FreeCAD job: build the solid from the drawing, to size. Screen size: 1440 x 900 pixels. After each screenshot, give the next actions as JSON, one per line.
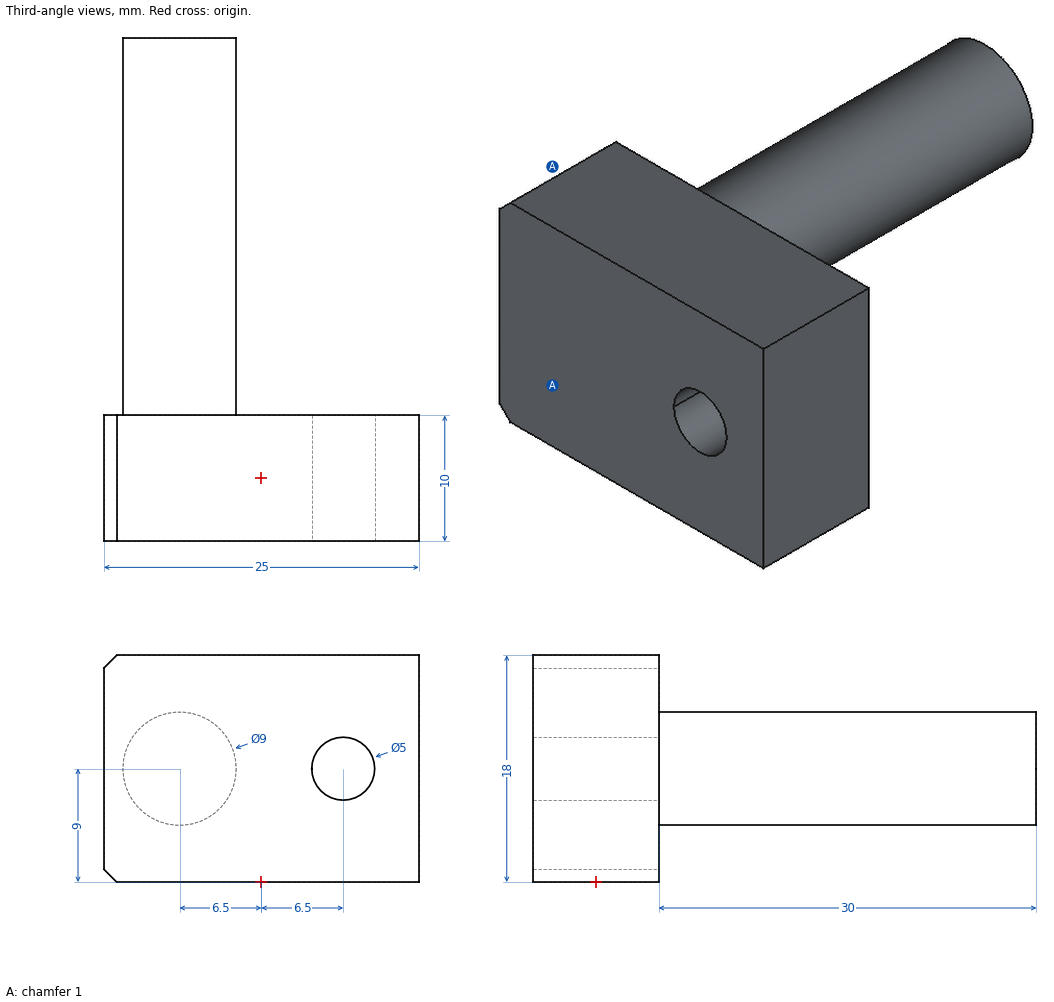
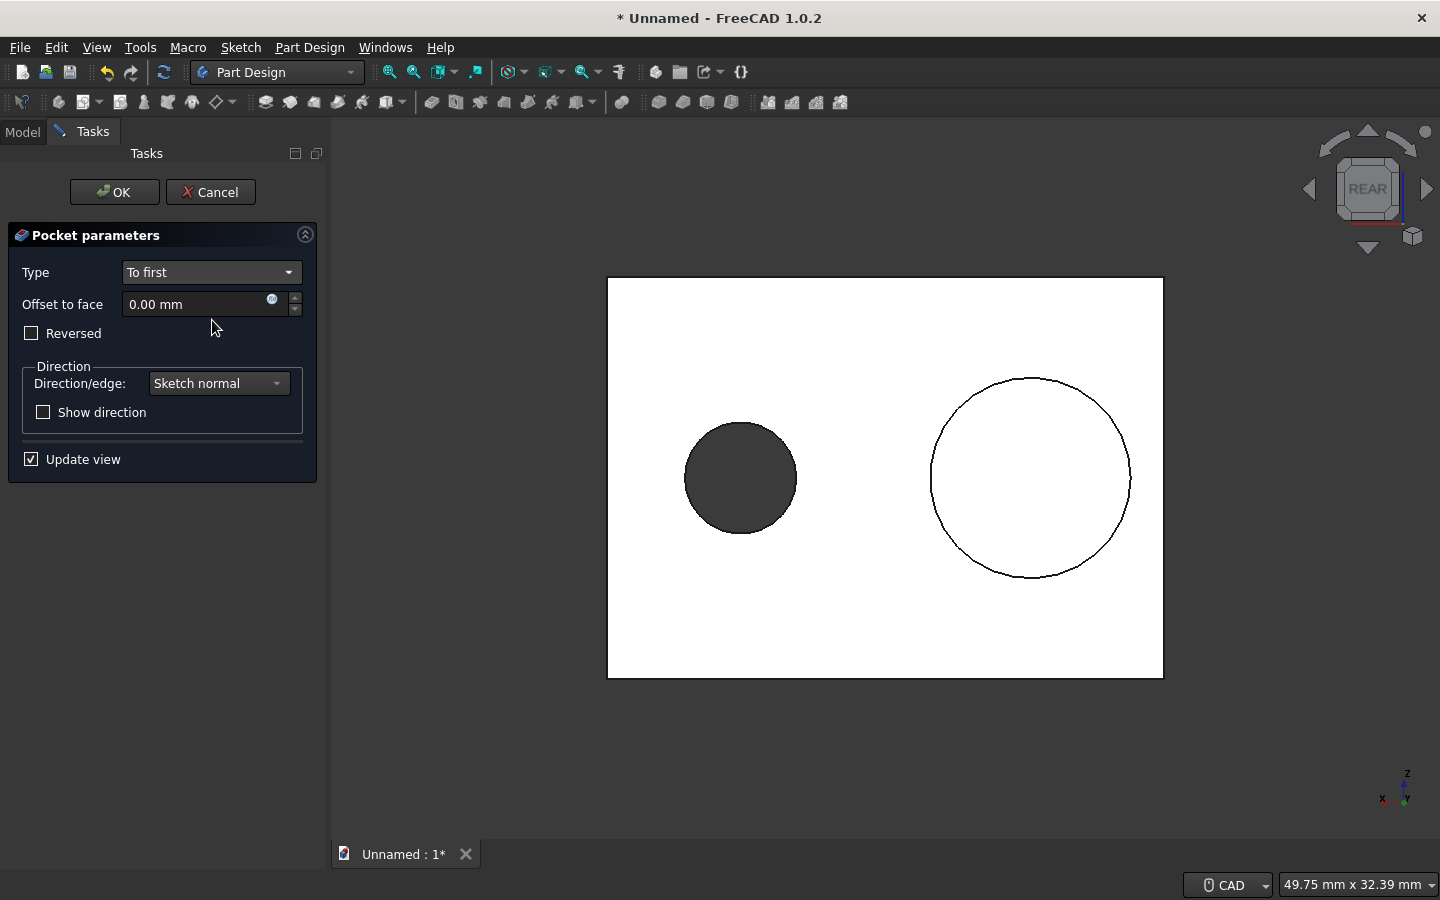
{"action": "left_click", "coordinate": [115, 192]}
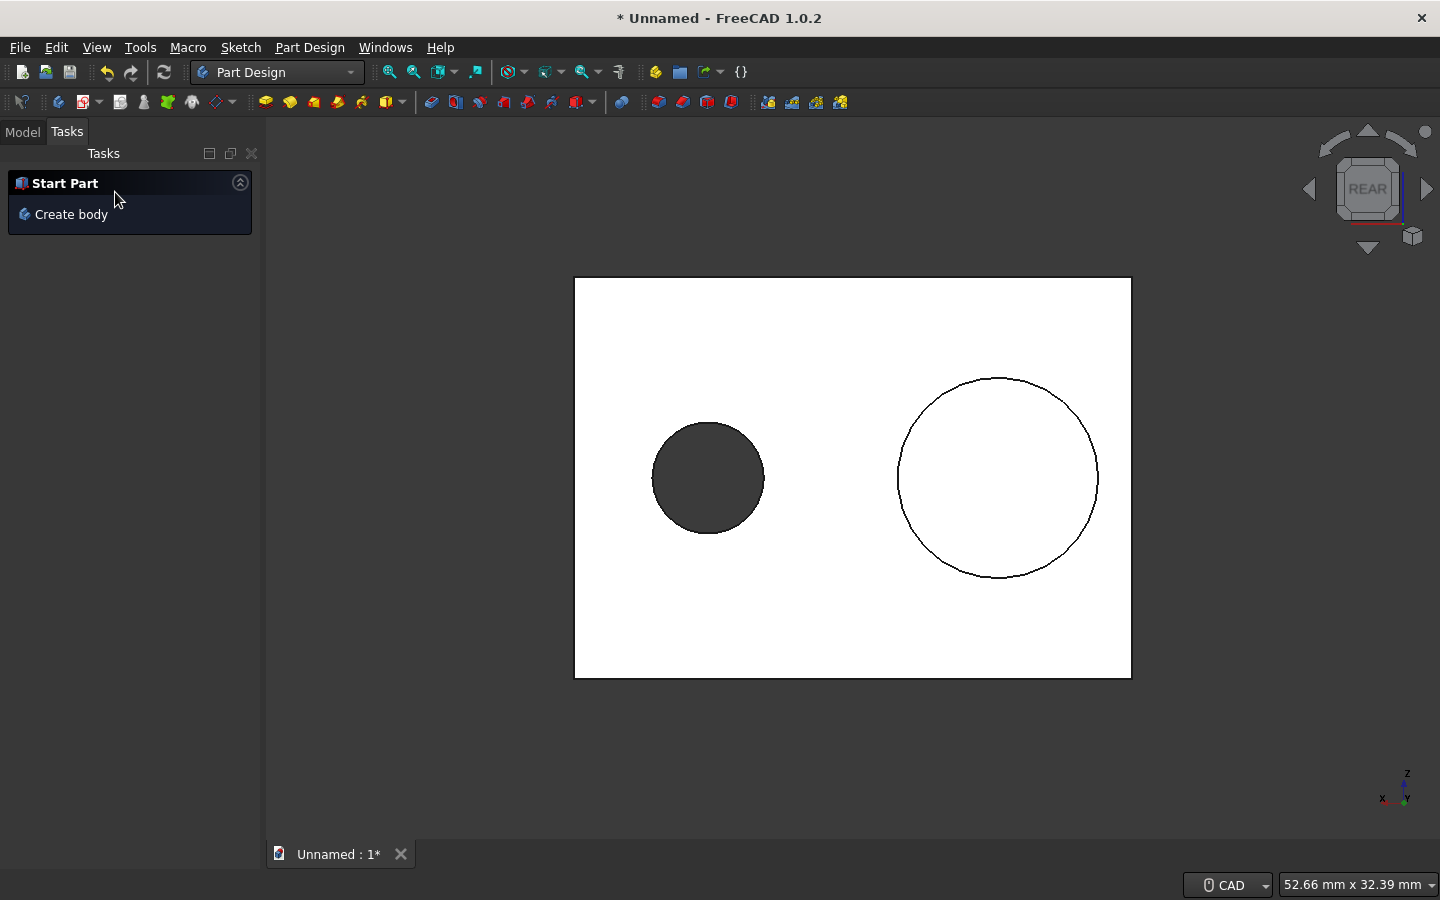
{"action": "key", "text": "0"}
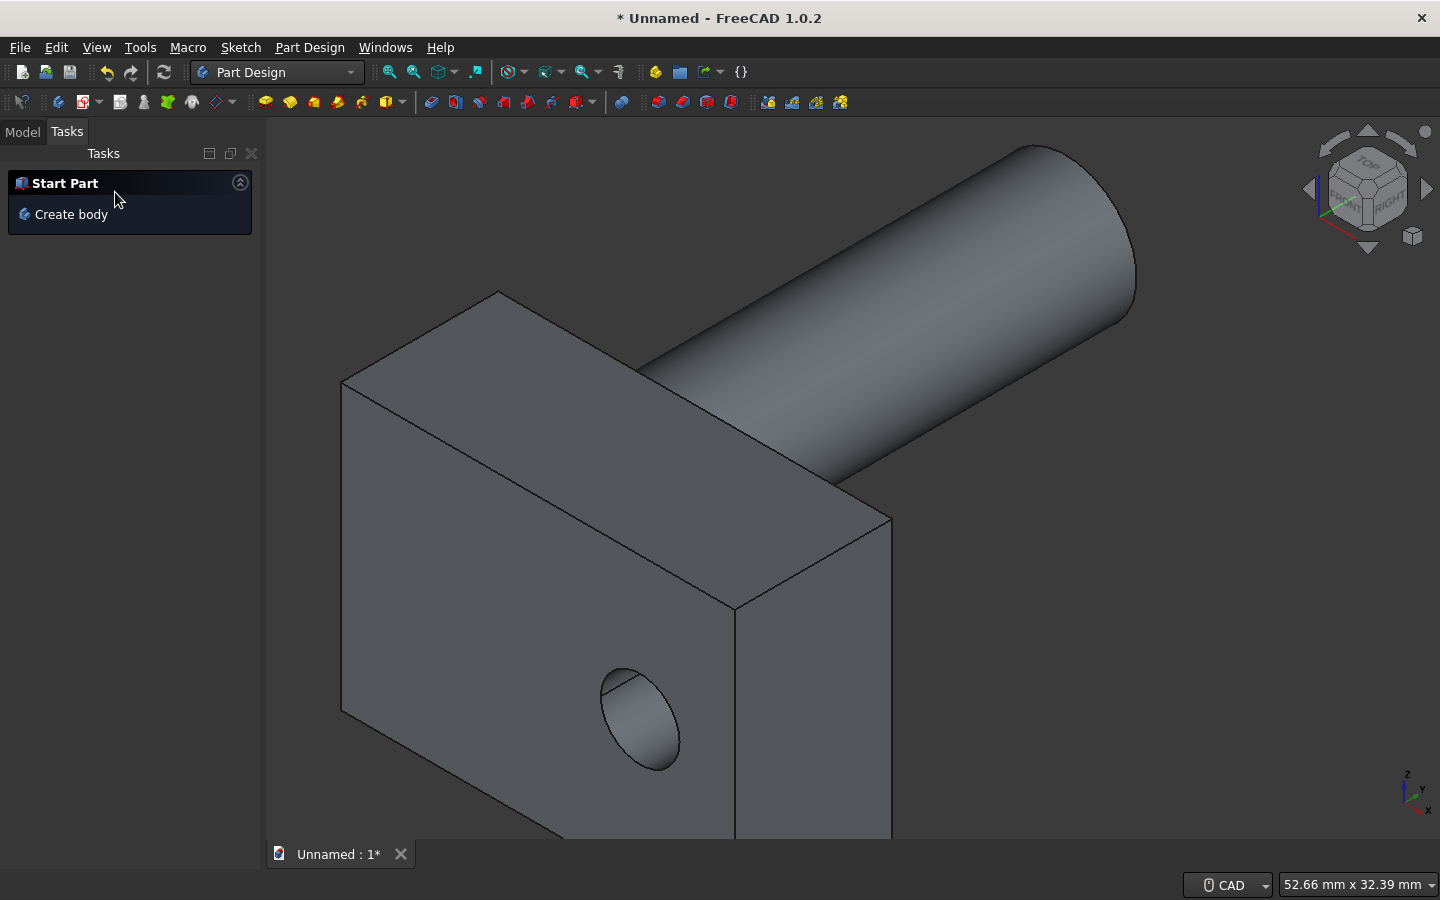
{"action": "key", "text": "v f"}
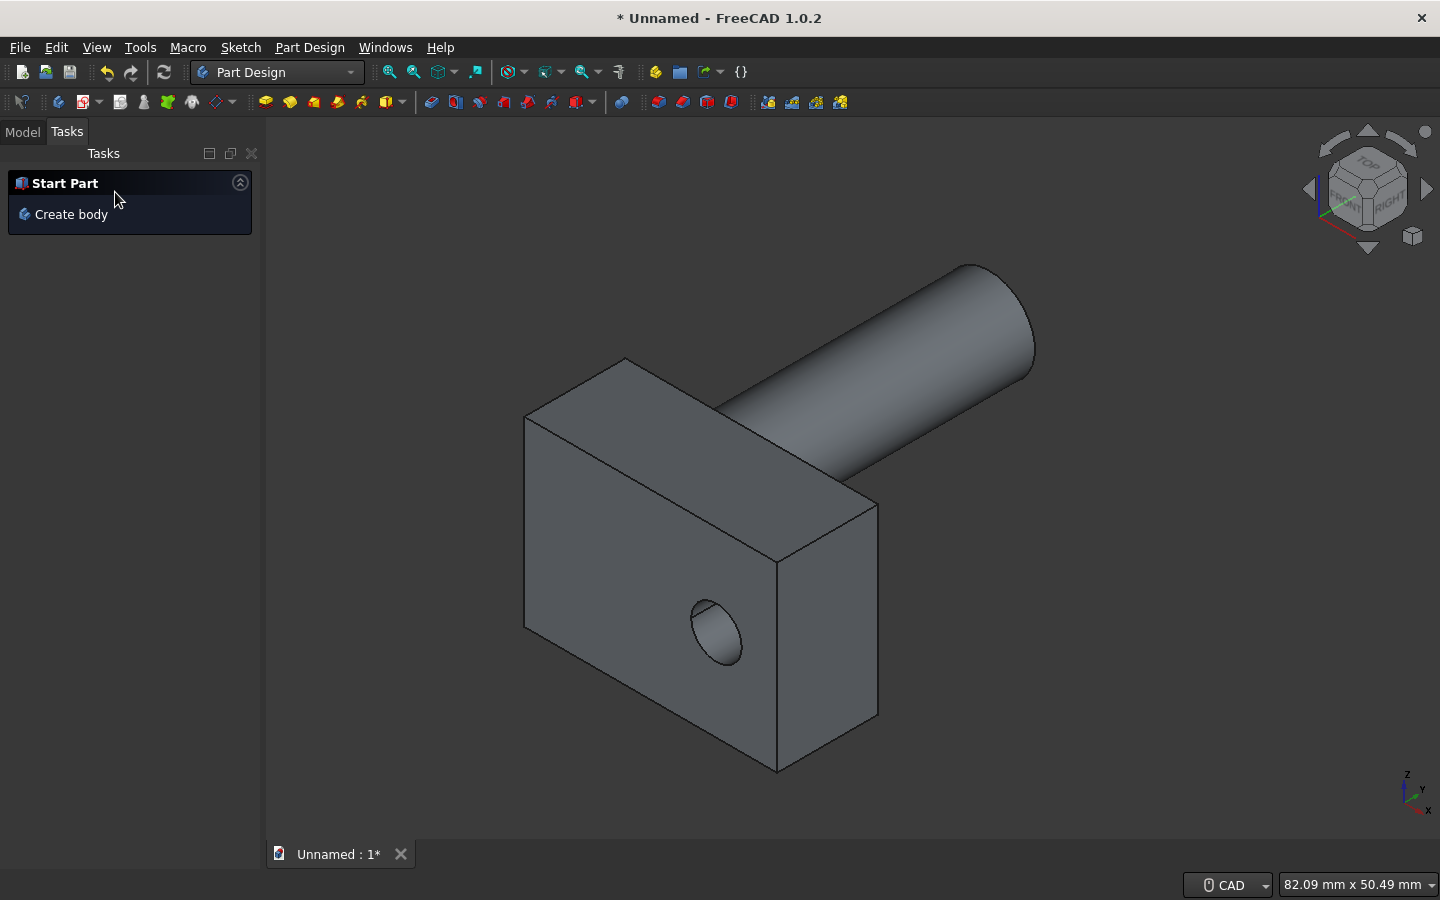
{"action": "key", "text": "2"}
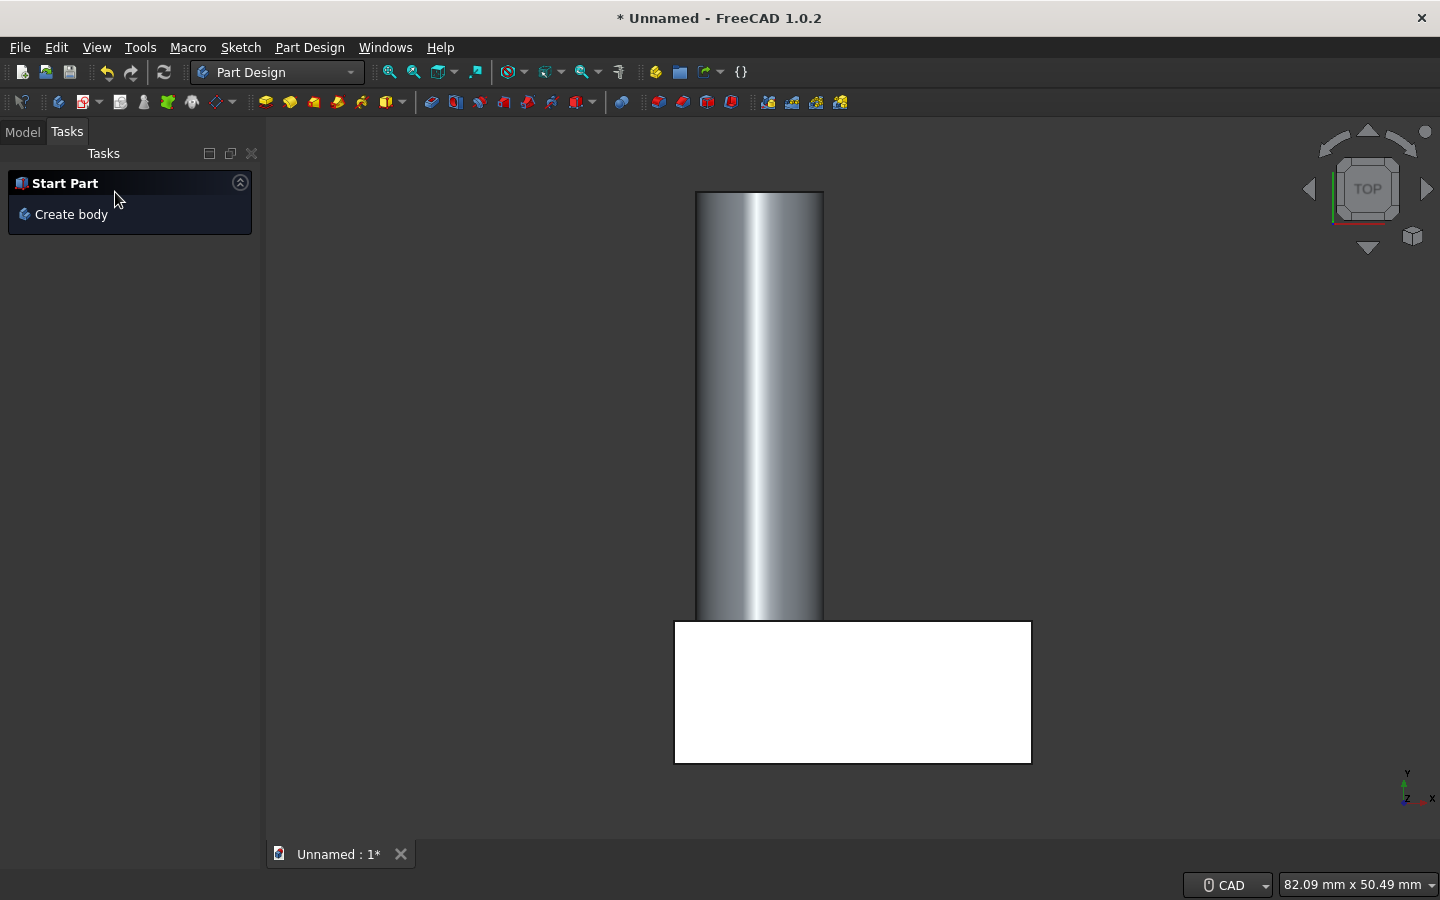
{"action": "left_click", "coordinate": [674, 692]}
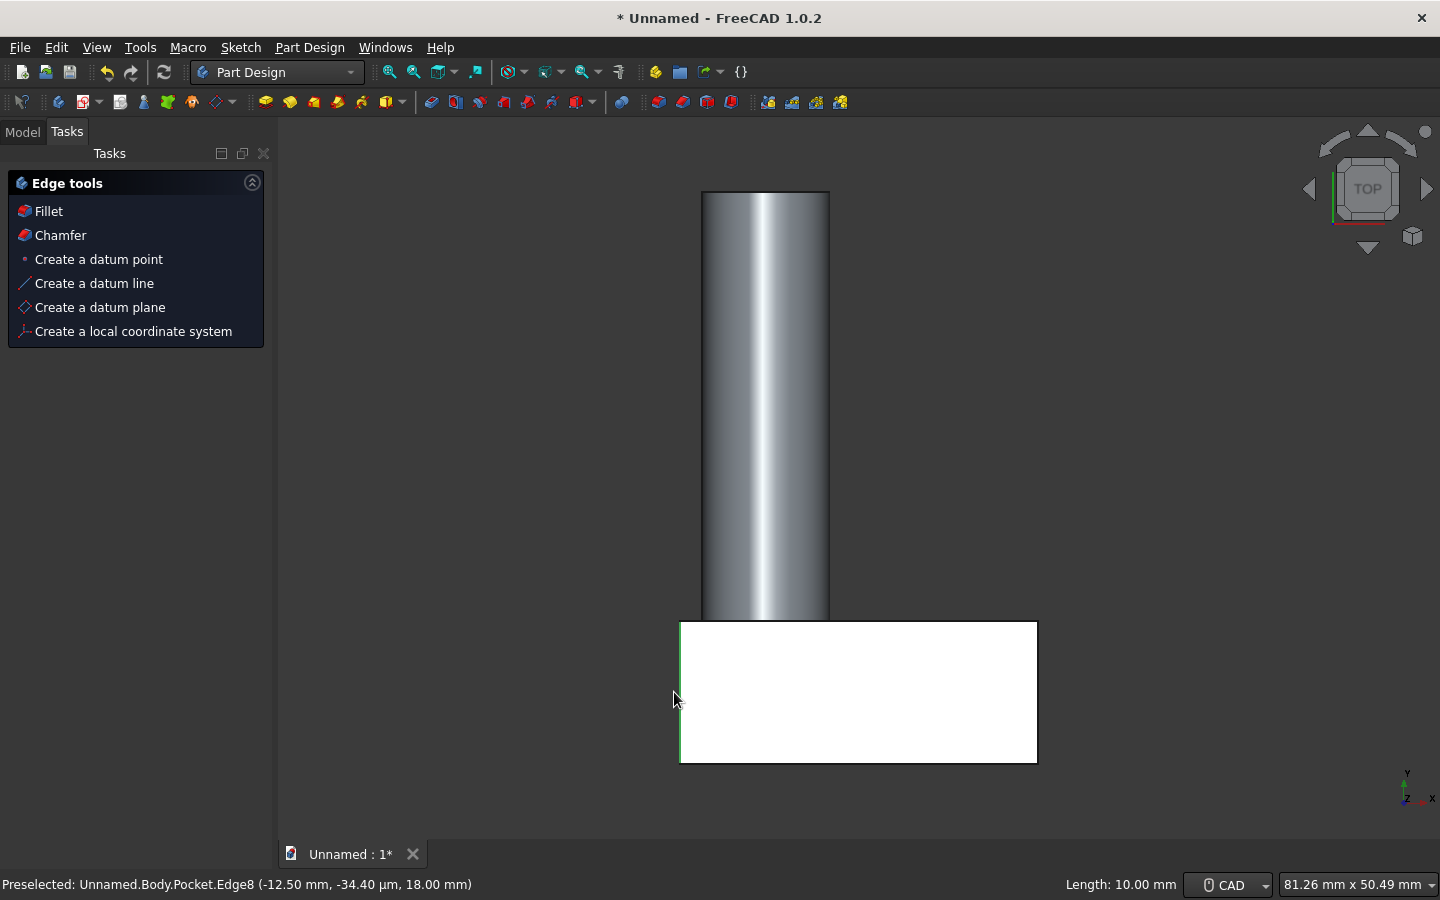
{"action": "key", "text": "1"}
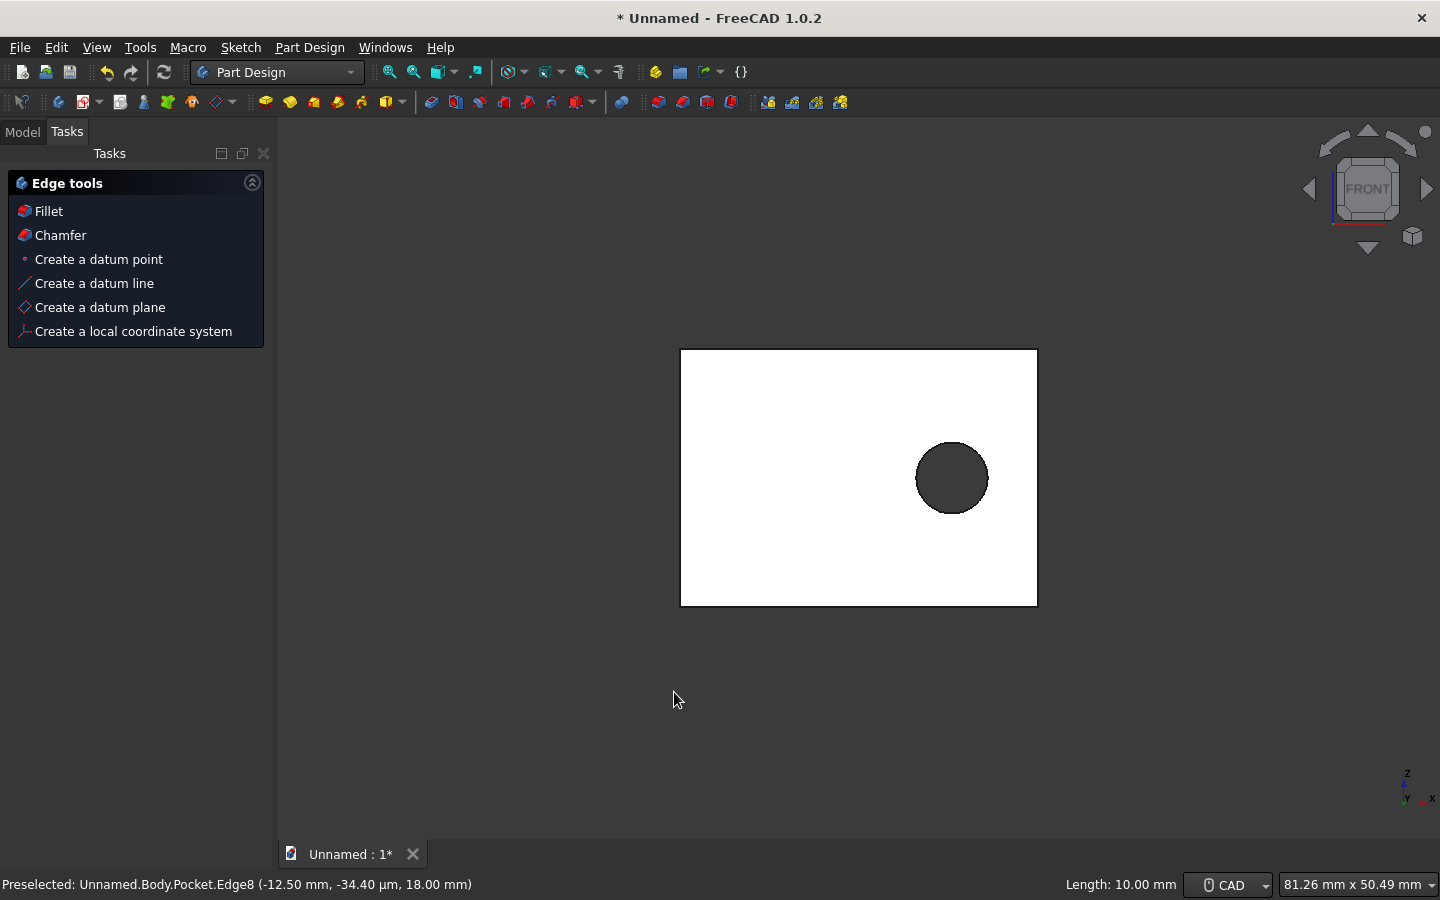
{"action": "key", "text": "v f"}